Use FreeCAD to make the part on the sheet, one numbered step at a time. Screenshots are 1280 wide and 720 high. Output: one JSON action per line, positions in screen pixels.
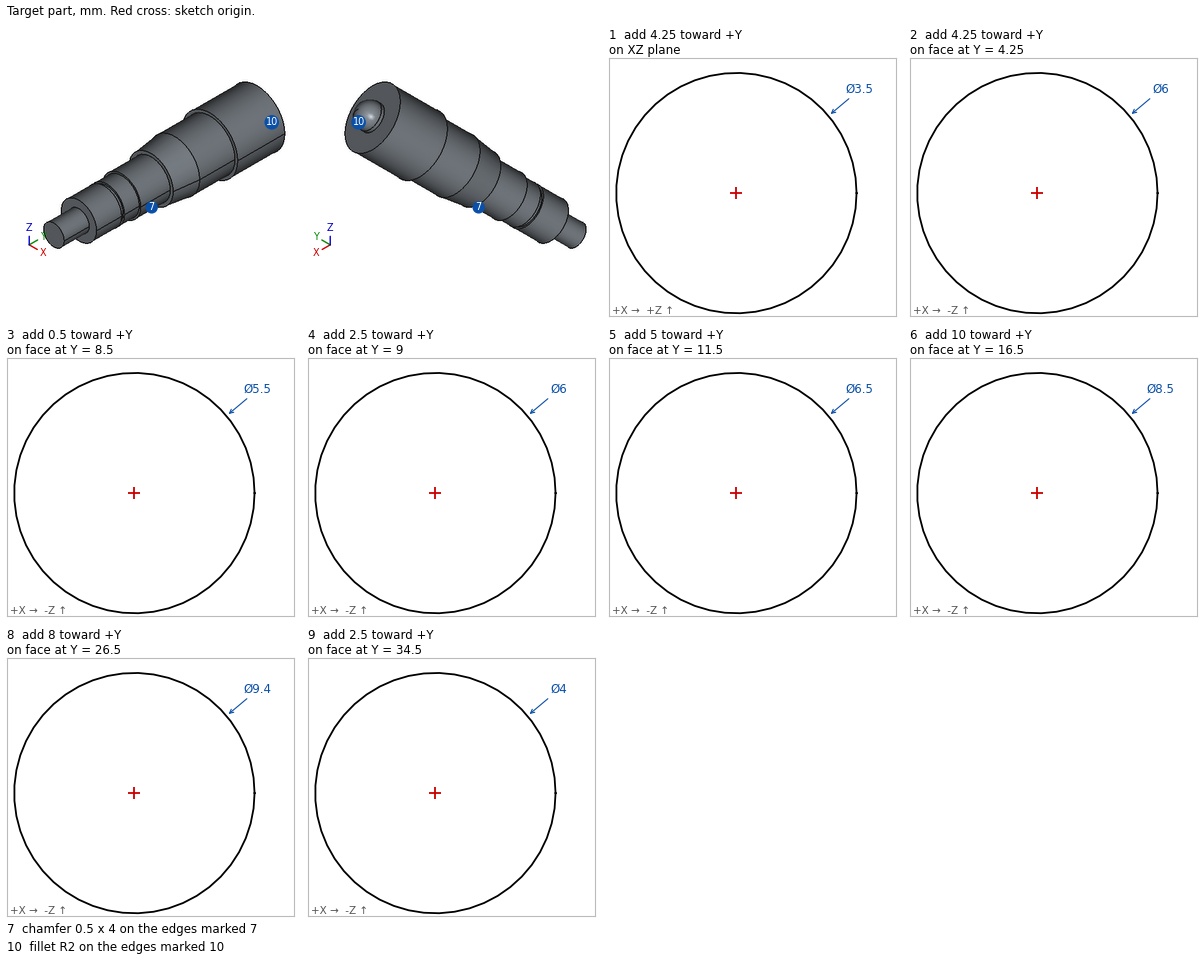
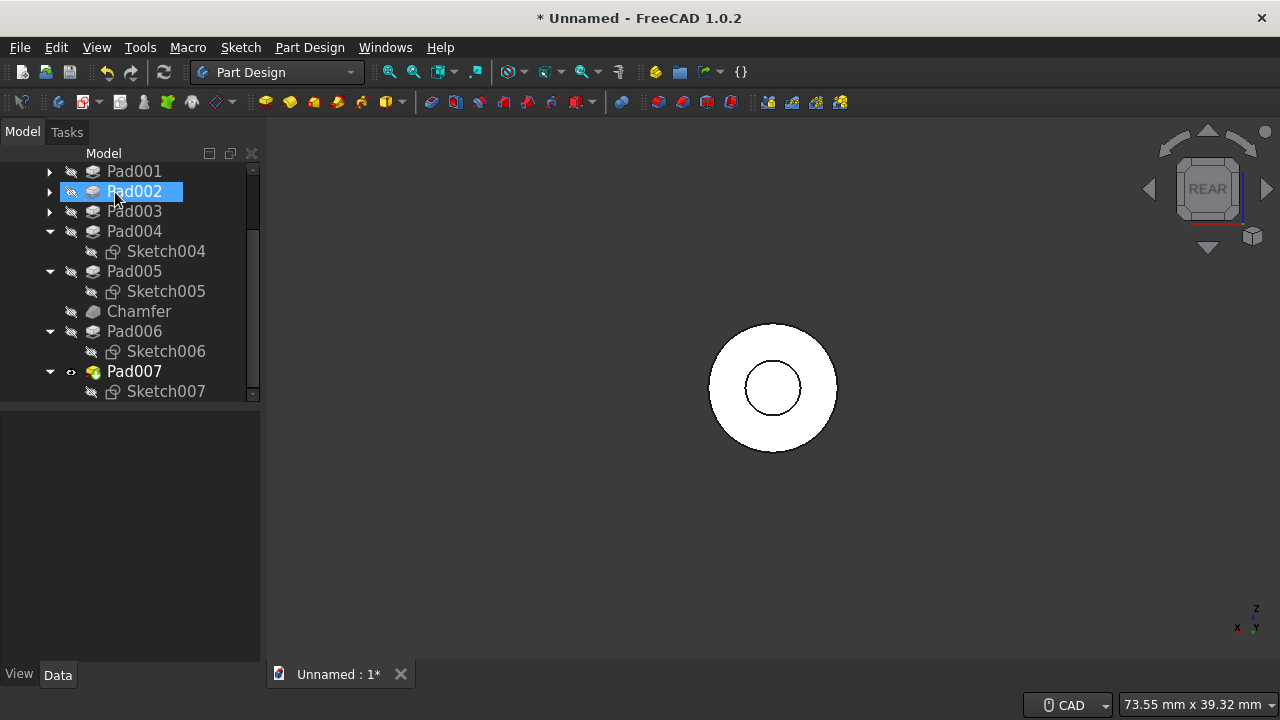
{"action": "left_click", "coordinate": [801, 387]}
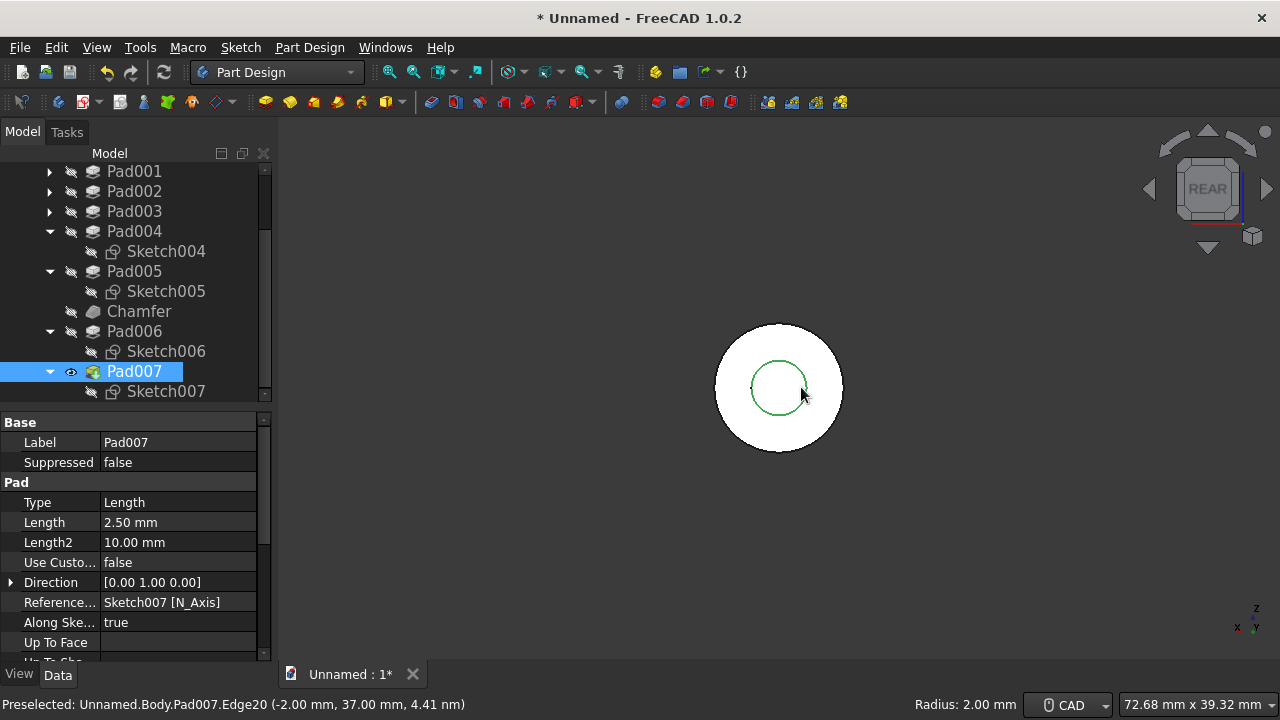
{"action": "left_click", "coordinate": [660, 102]}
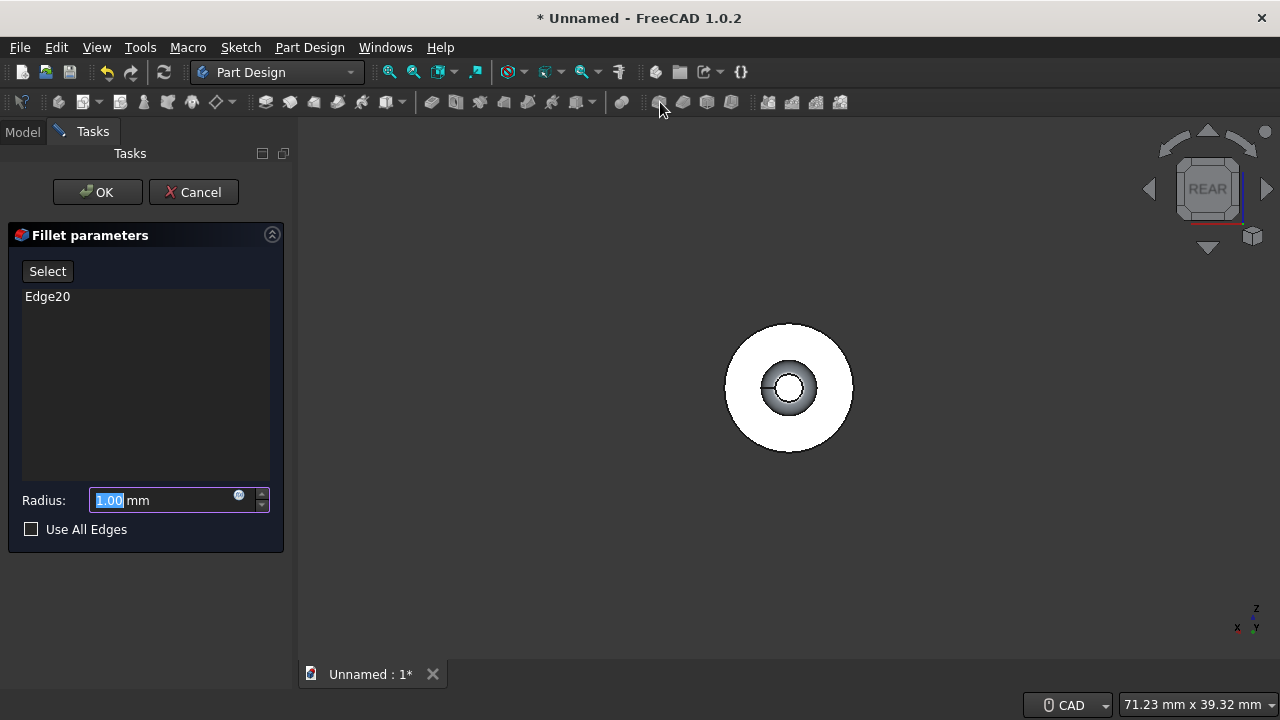
{"action": "type", "text": "2"}
{"action": "key", "text": "Tab"}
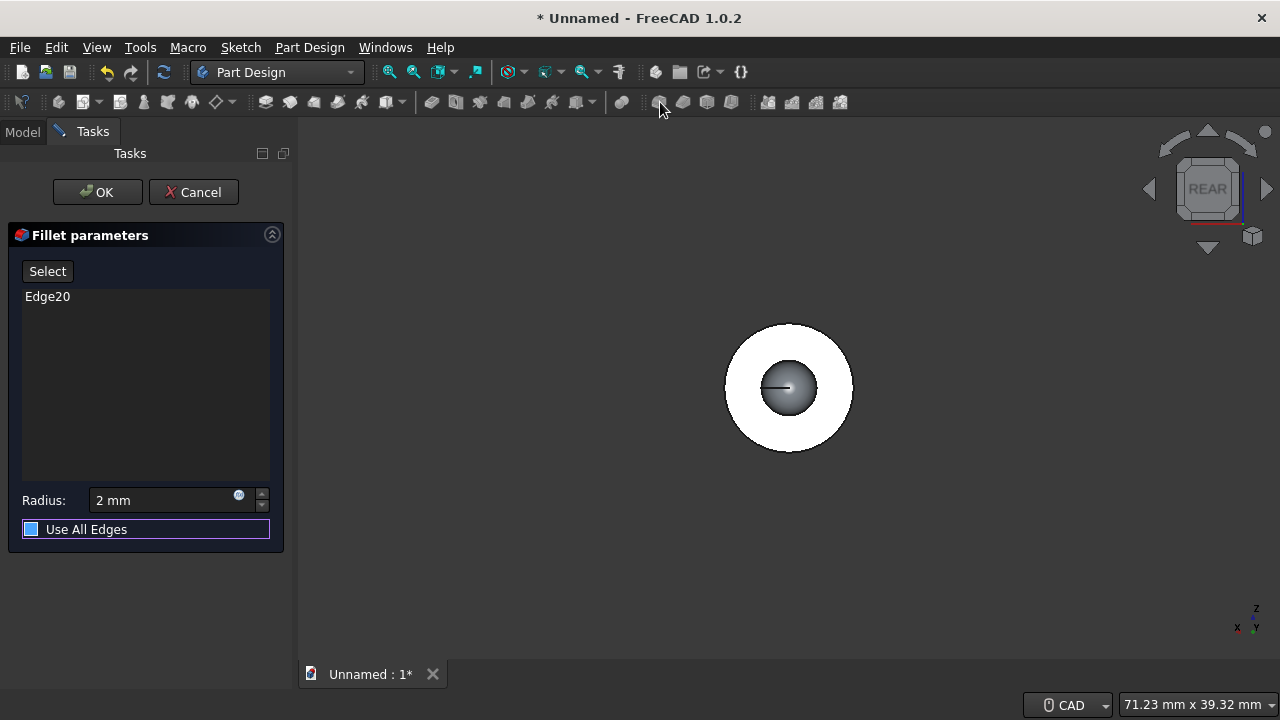
{"action": "left_click", "coordinate": [98, 192]}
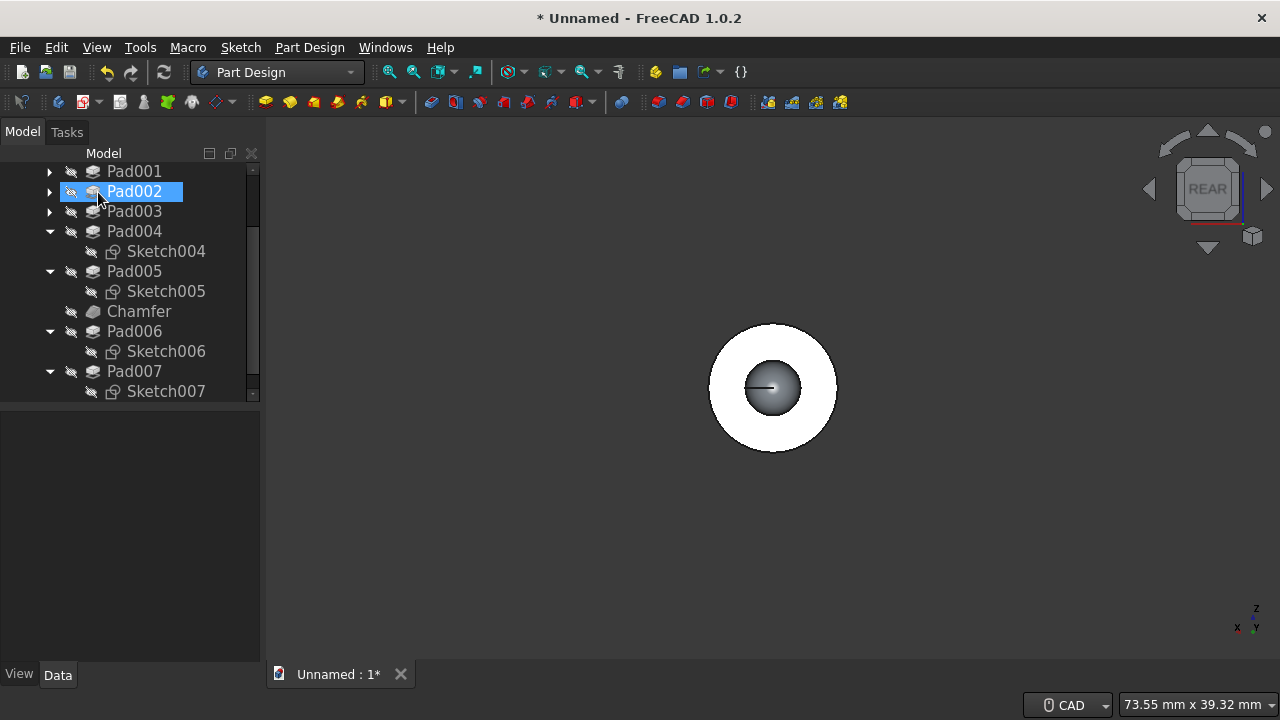
{"action": "key", "text": "0"}